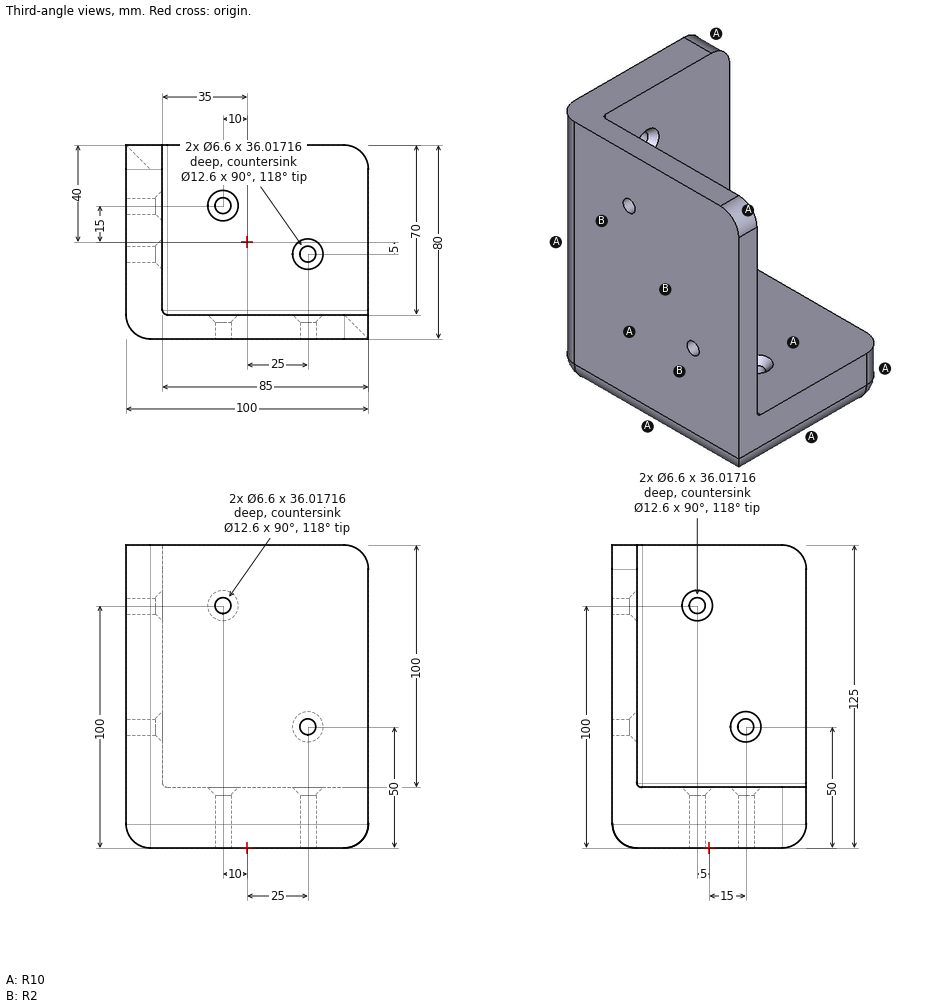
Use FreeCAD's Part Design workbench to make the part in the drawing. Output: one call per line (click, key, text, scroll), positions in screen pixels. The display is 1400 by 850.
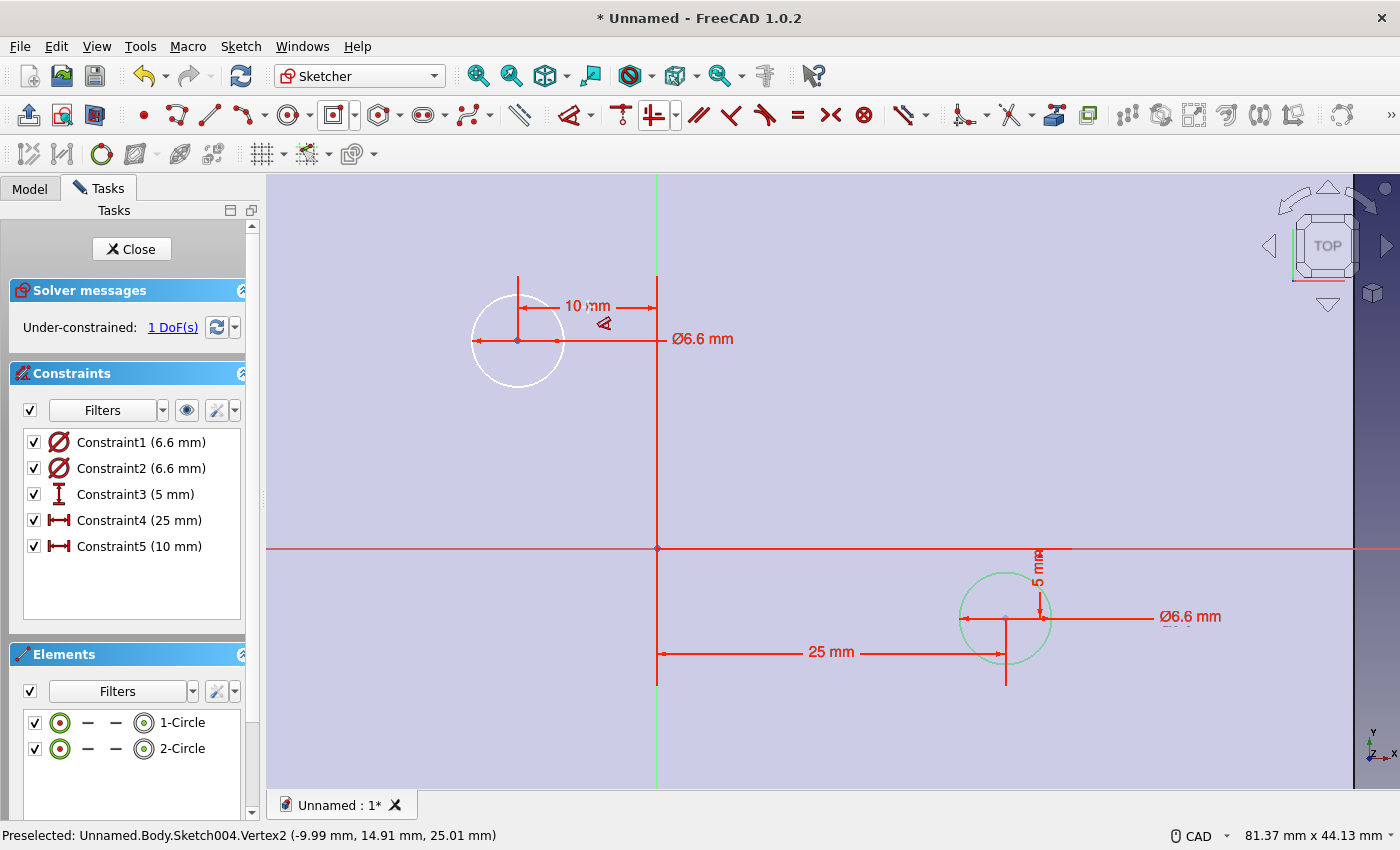
click(518, 341)
click(484, 445)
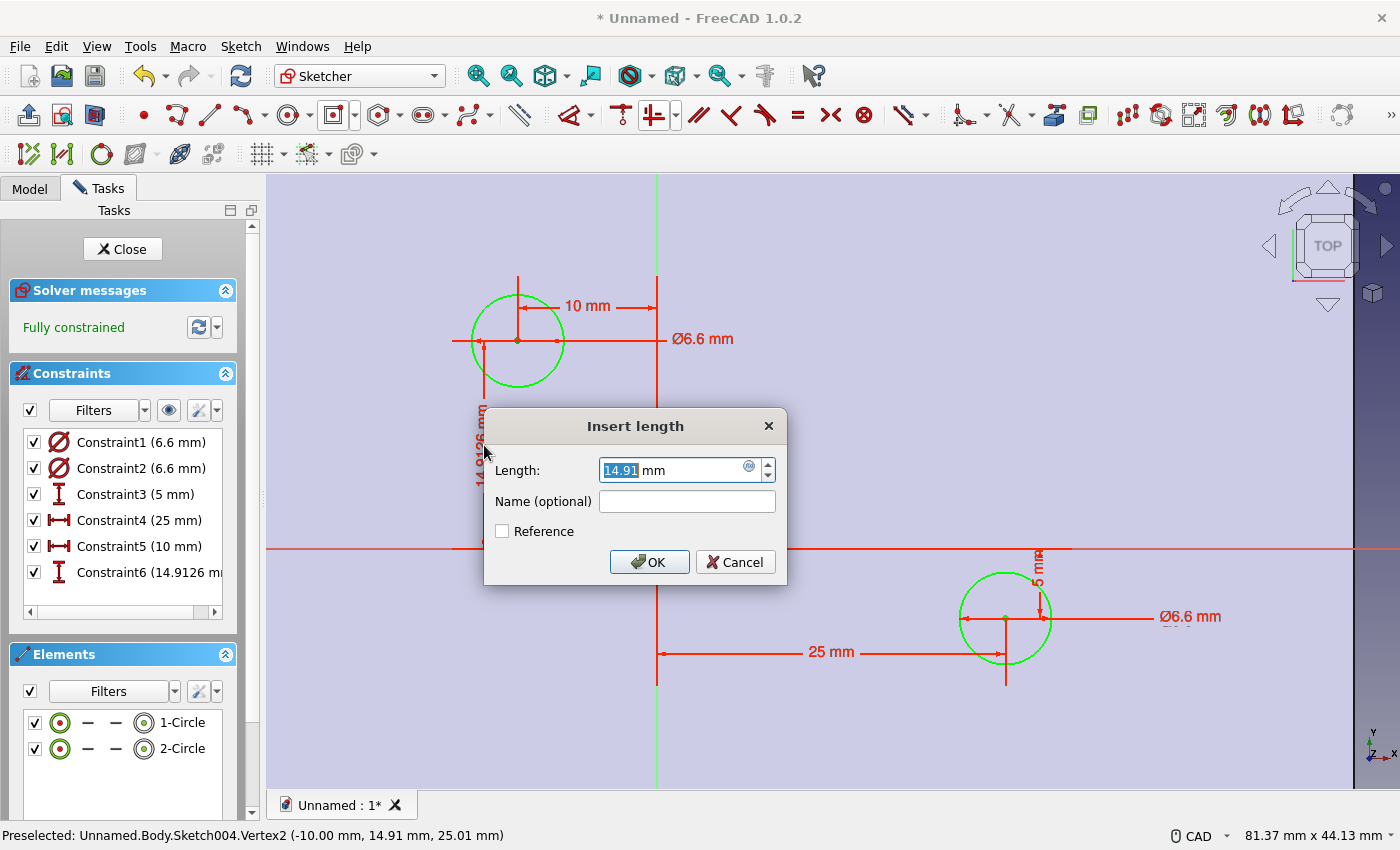
text(15)
key(Return)
key(Escape)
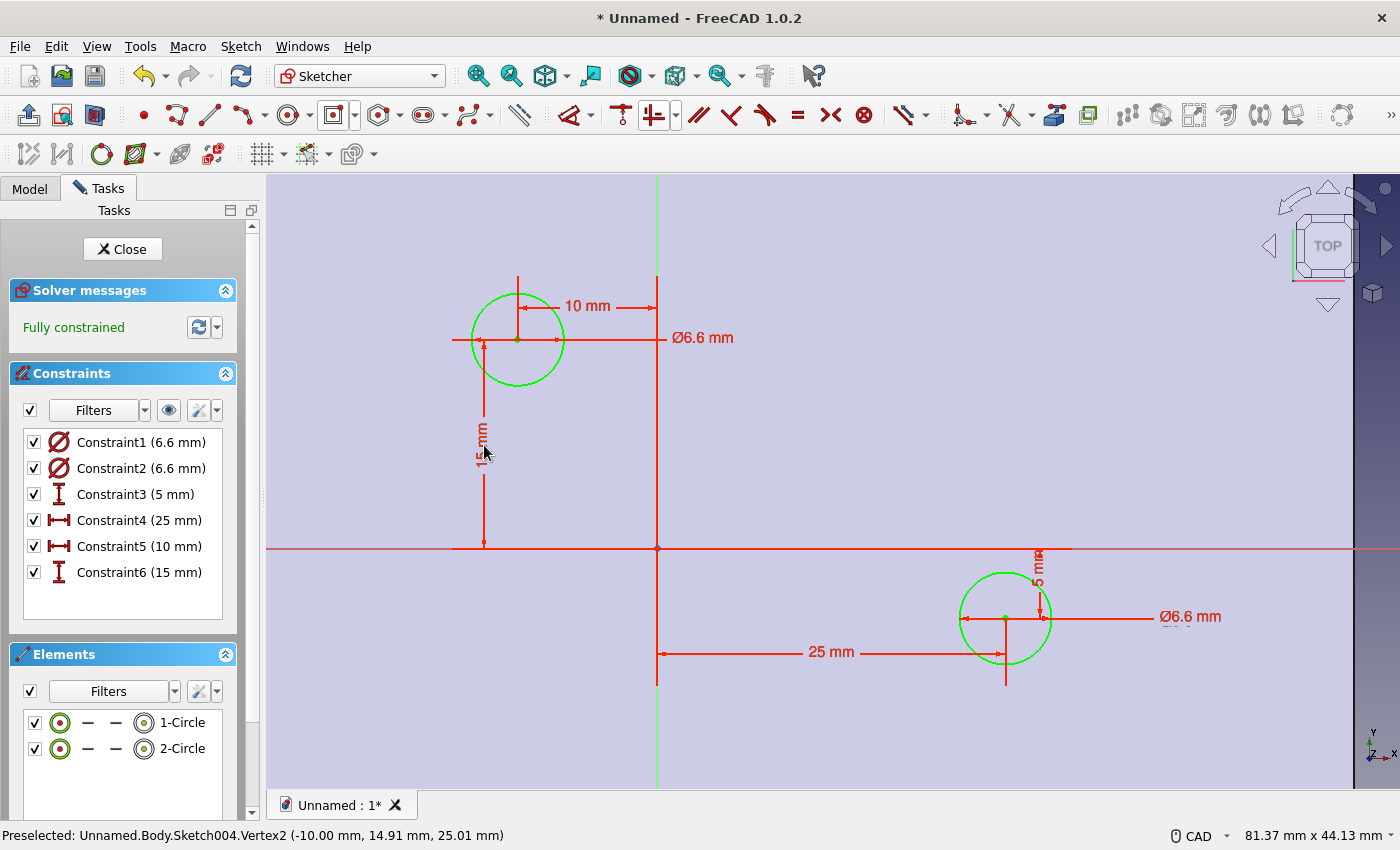
click(123, 249)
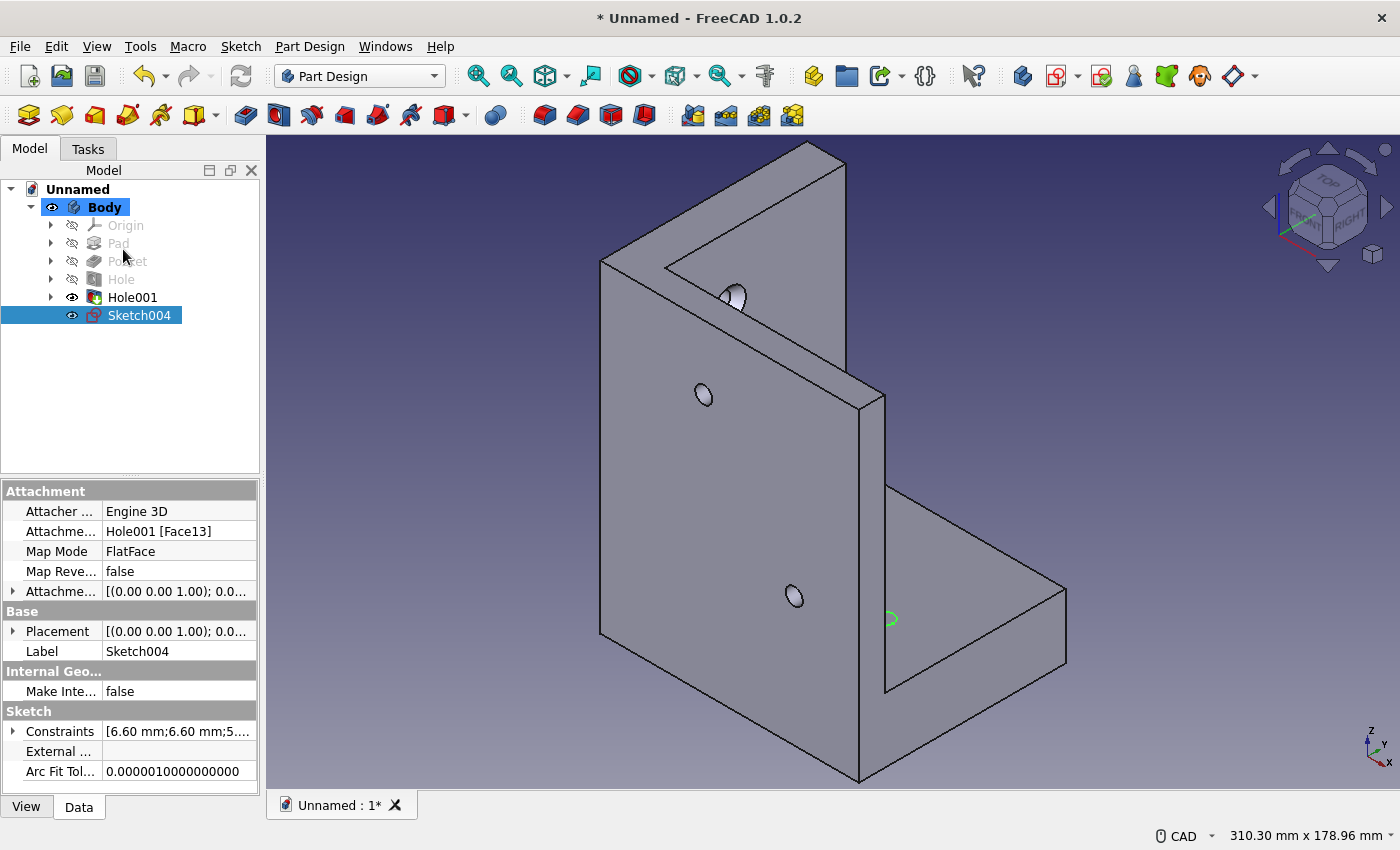
click(279, 116)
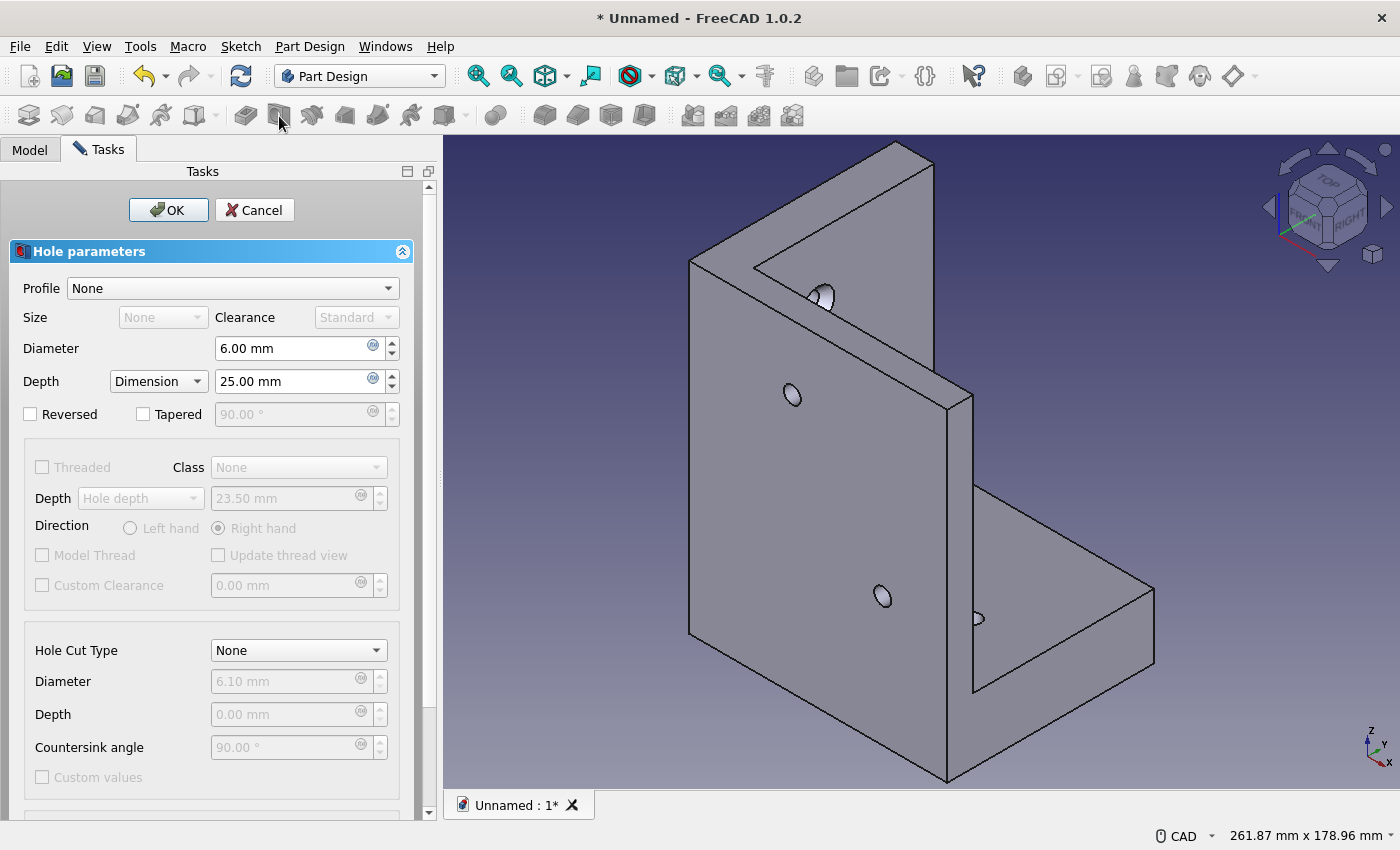
triple_click(300, 348)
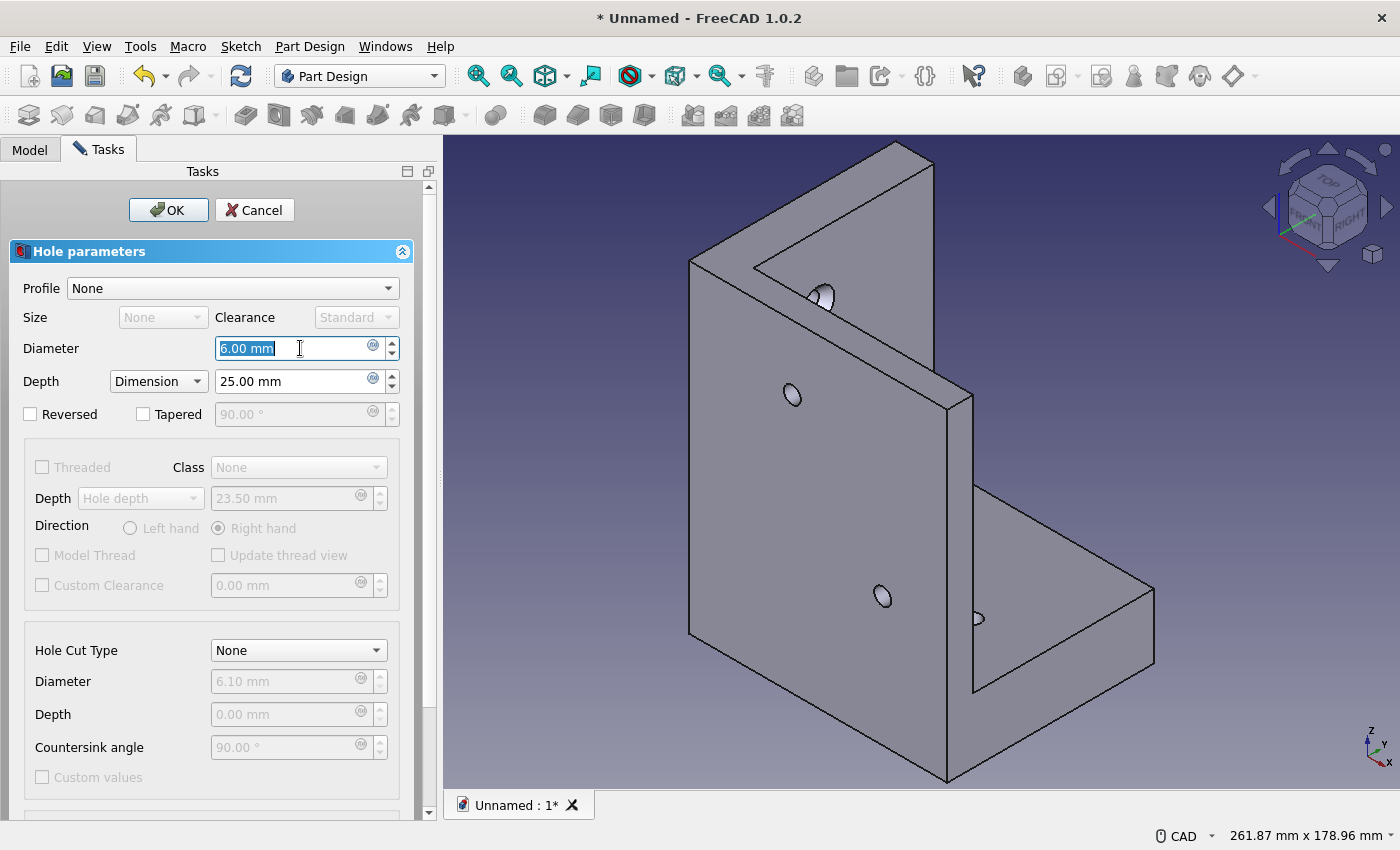
text(6.6)
key(Tab)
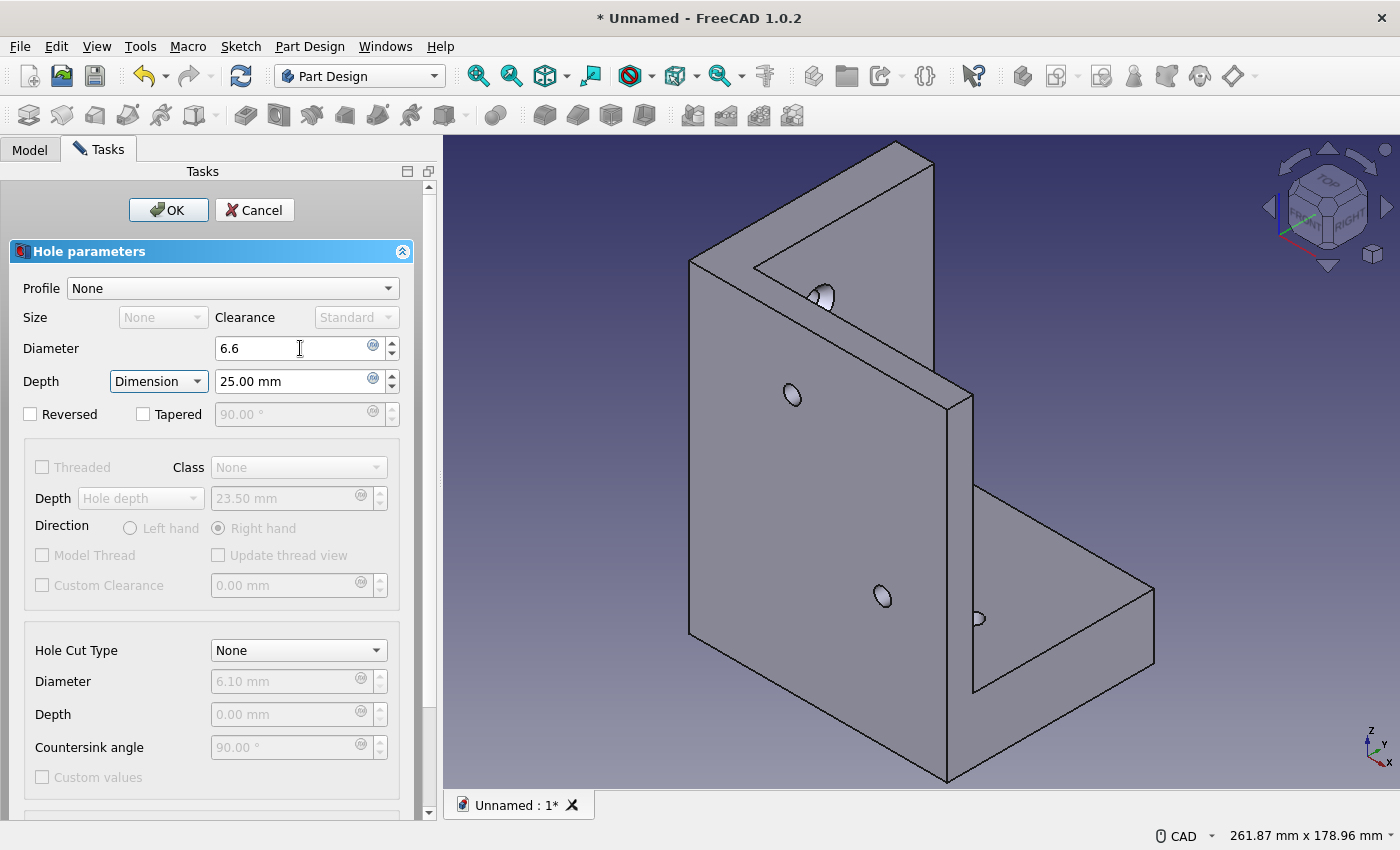
triple_click(300, 382)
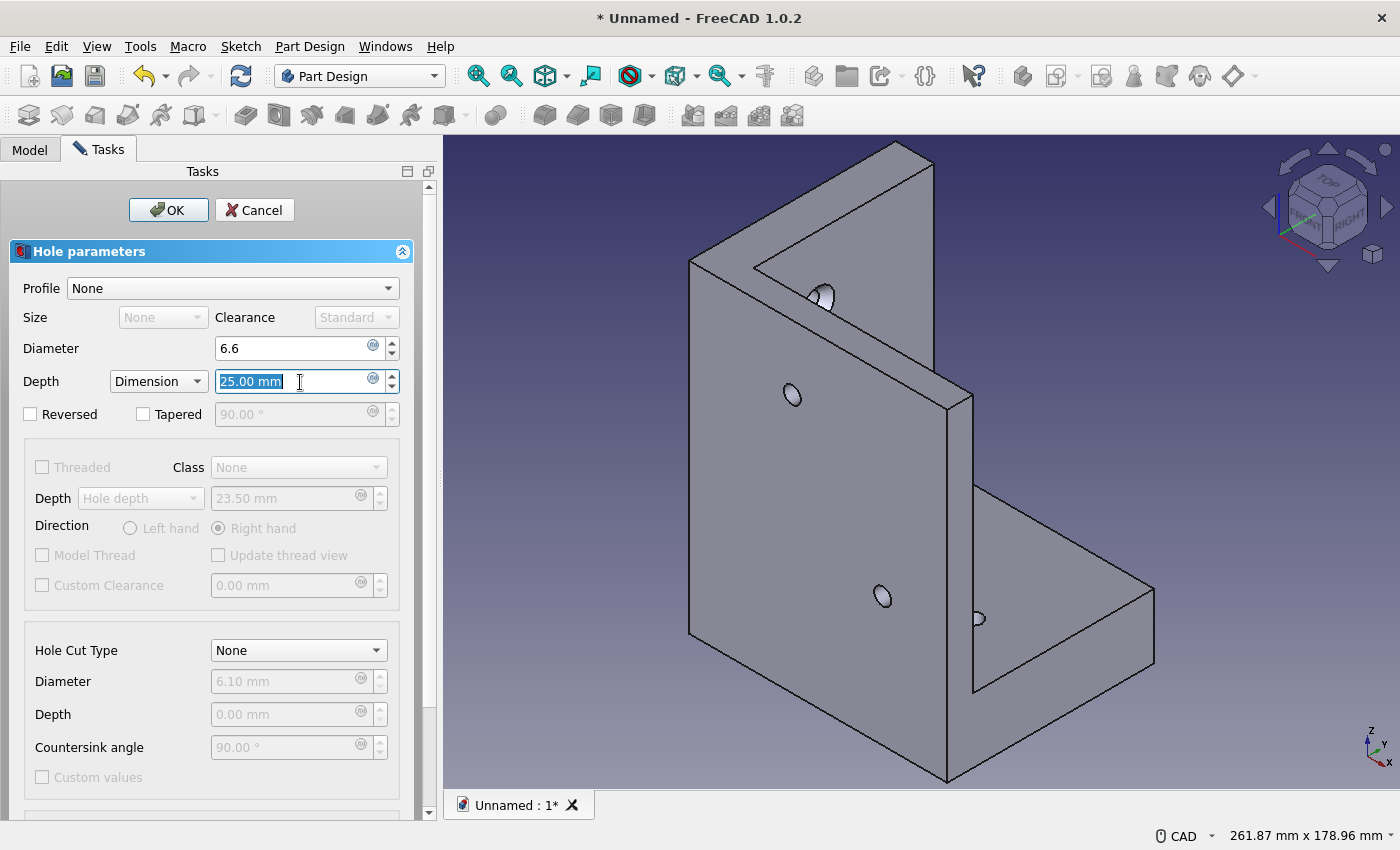
text(36.01716)
key(Tab)